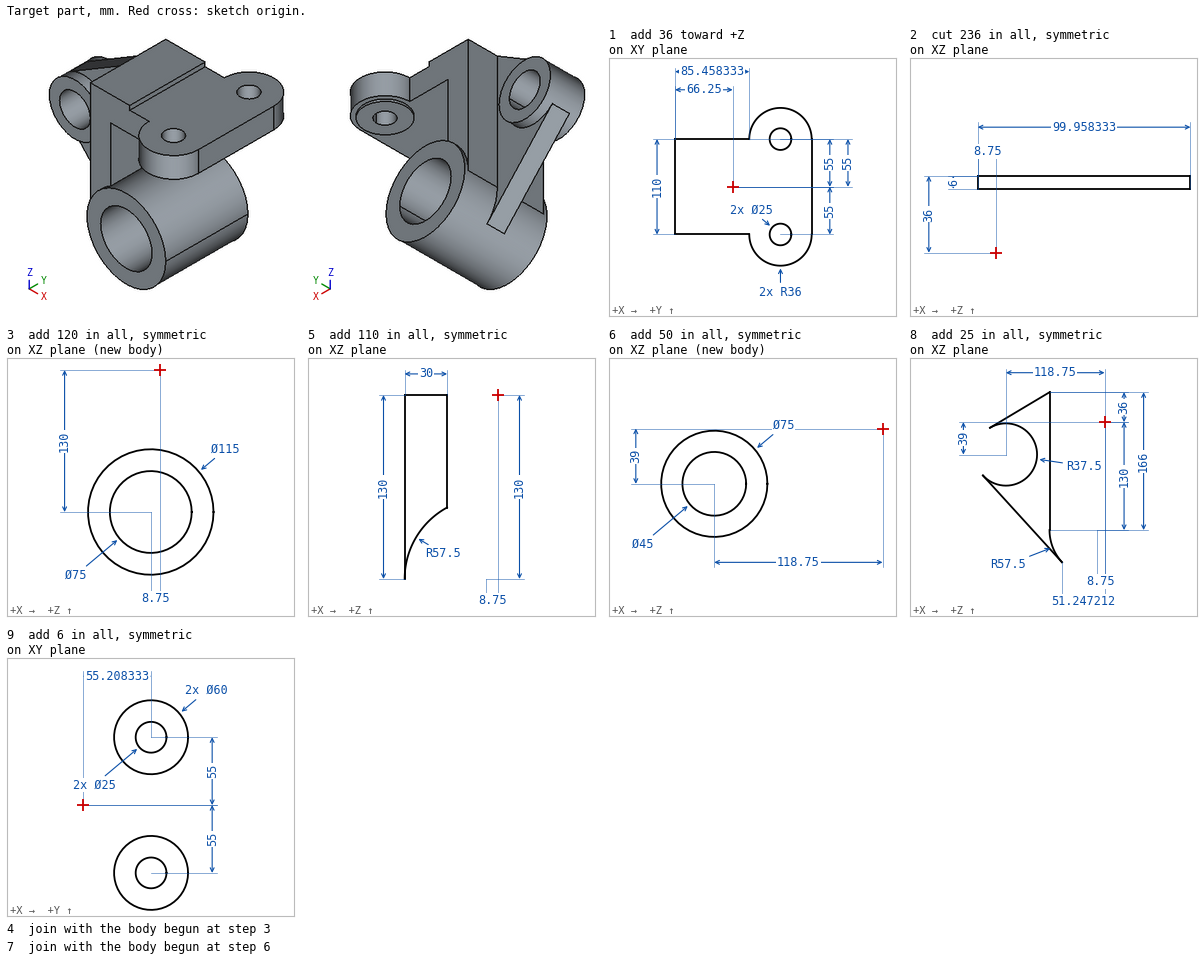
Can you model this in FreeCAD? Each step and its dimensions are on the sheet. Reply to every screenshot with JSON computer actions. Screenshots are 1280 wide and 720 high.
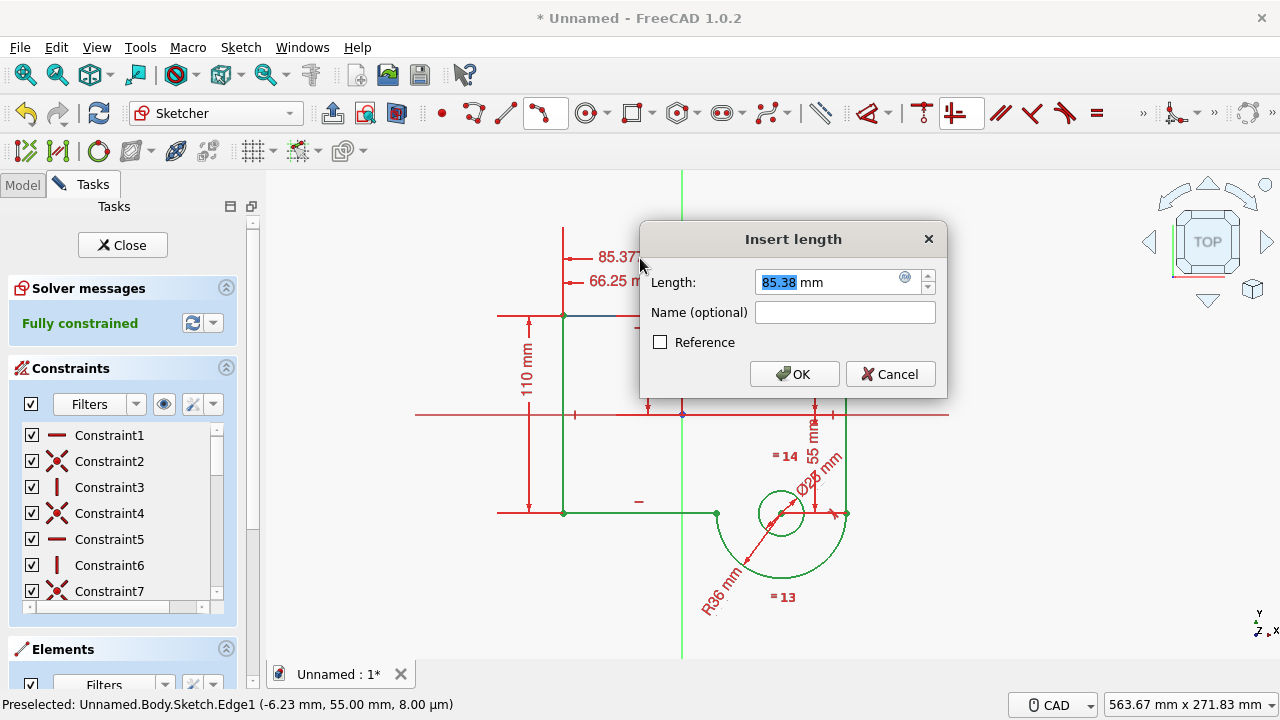
{"action": "type", "text": "85.458333"}
{"action": "key", "text": "Return"}
{"action": "key", "text": "Escape"}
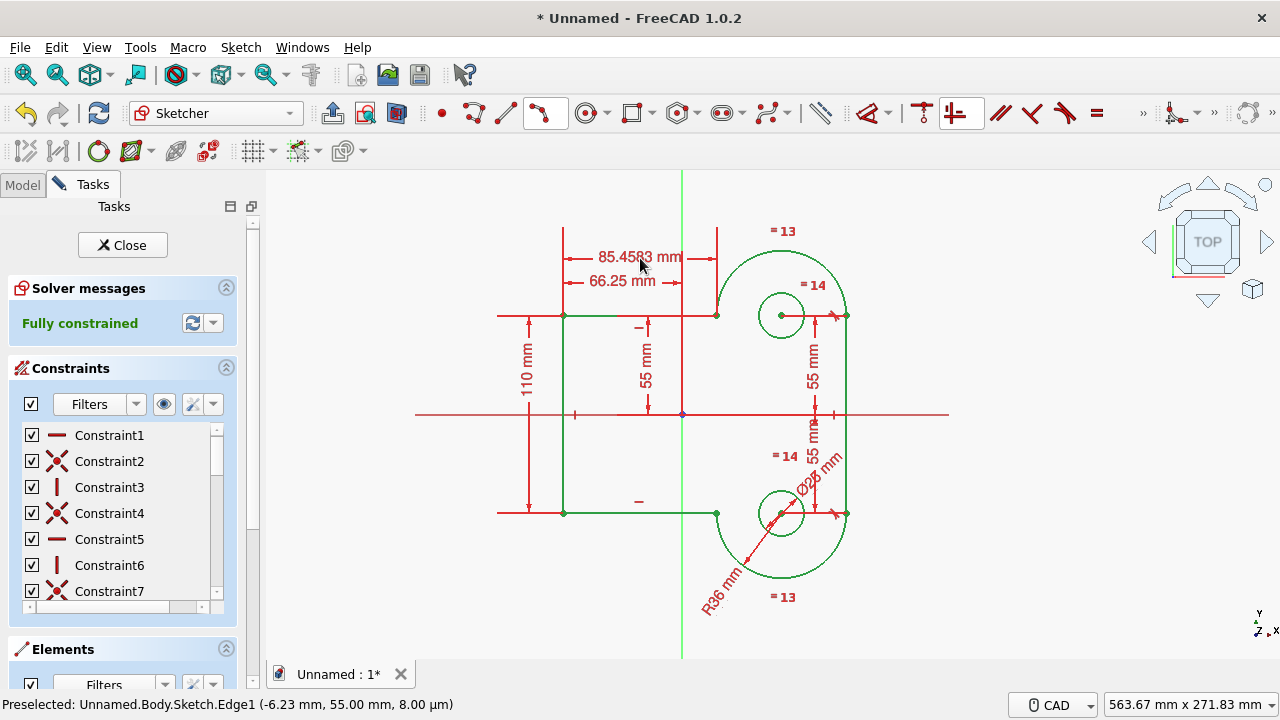
{"action": "left_click", "coordinate": [123, 245]}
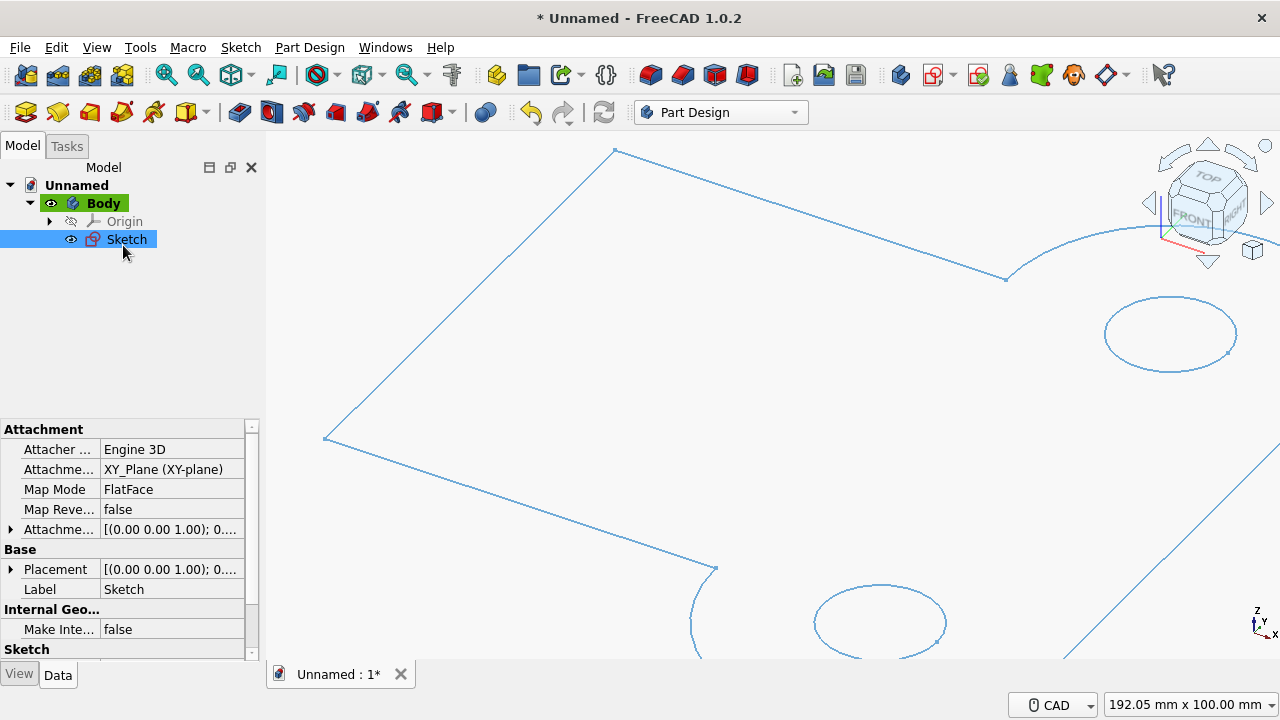
{"action": "left_click", "coordinate": [26, 112]}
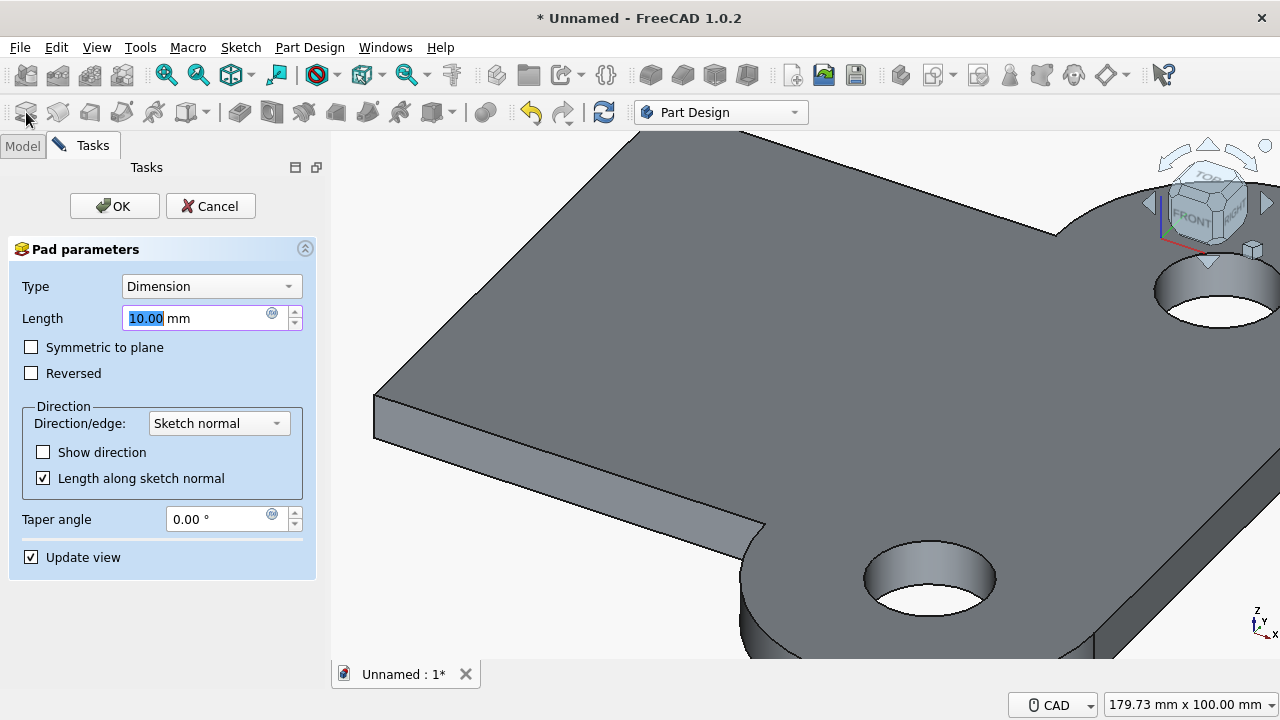
{"action": "type", "text": "36"}
{"action": "key", "text": "Tab"}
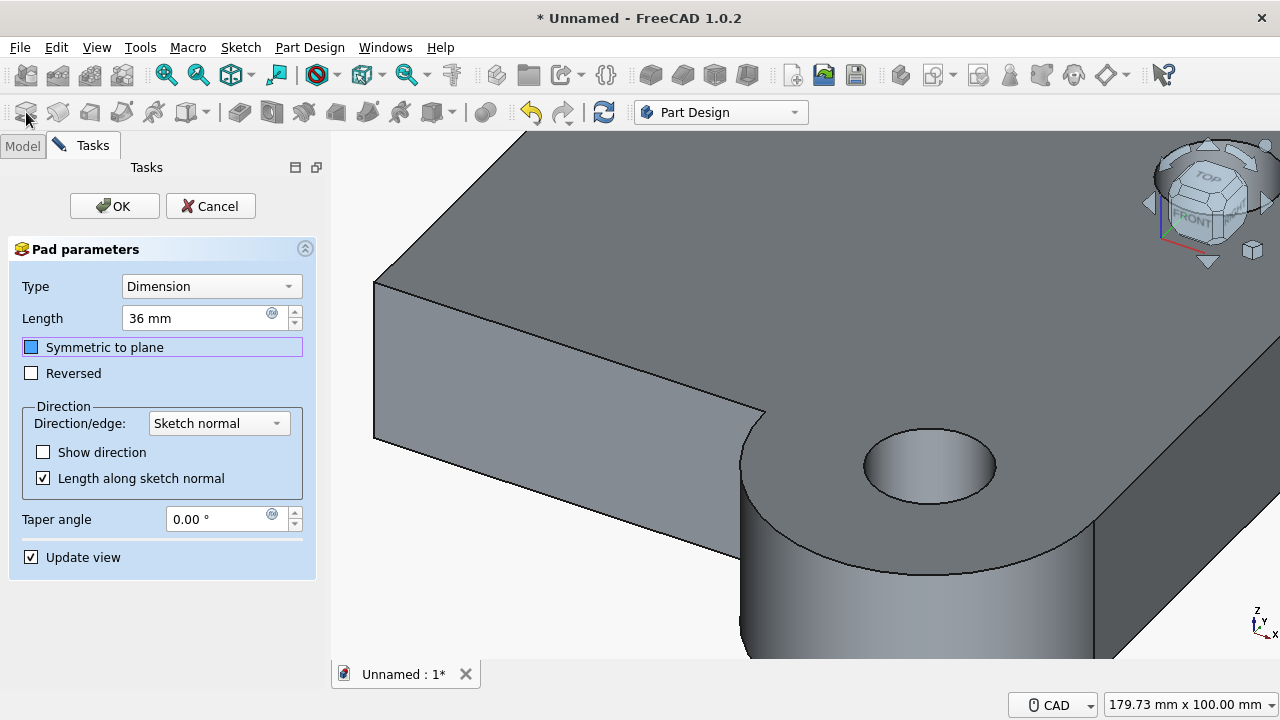
{"action": "left_click", "coordinate": [115, 206]}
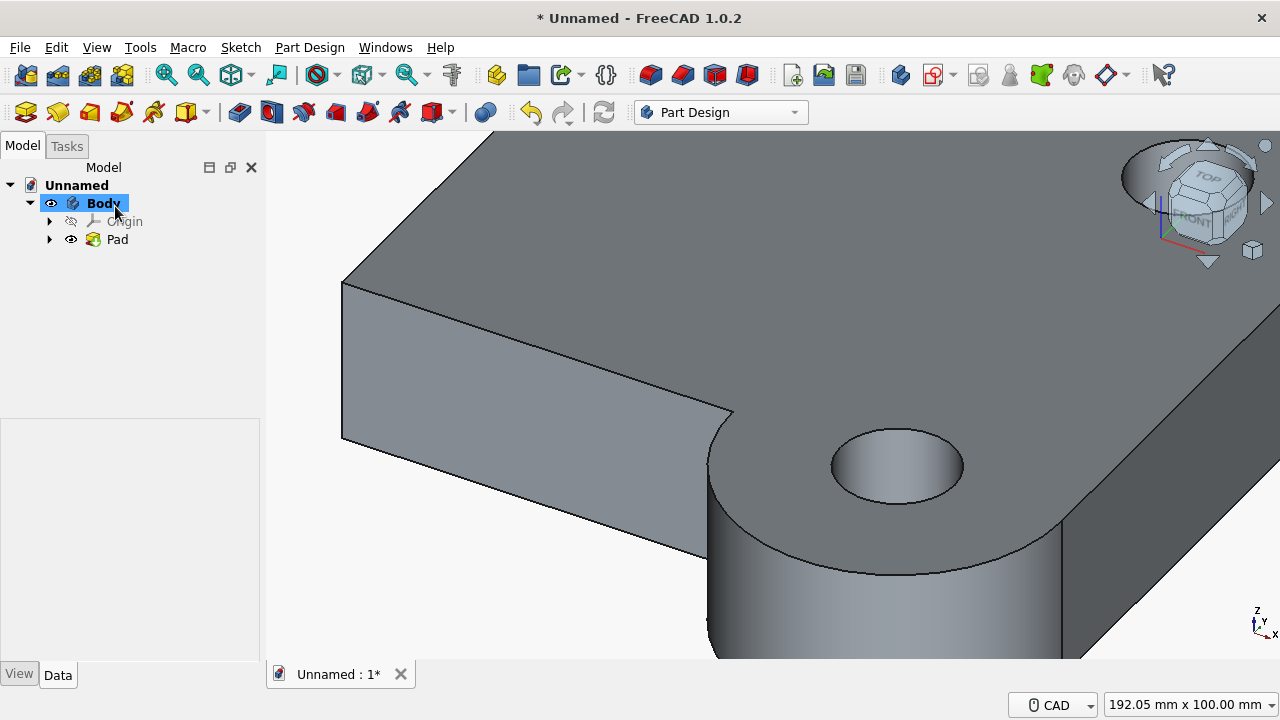
{"action": "left_click", "coordinate": [168, 76]}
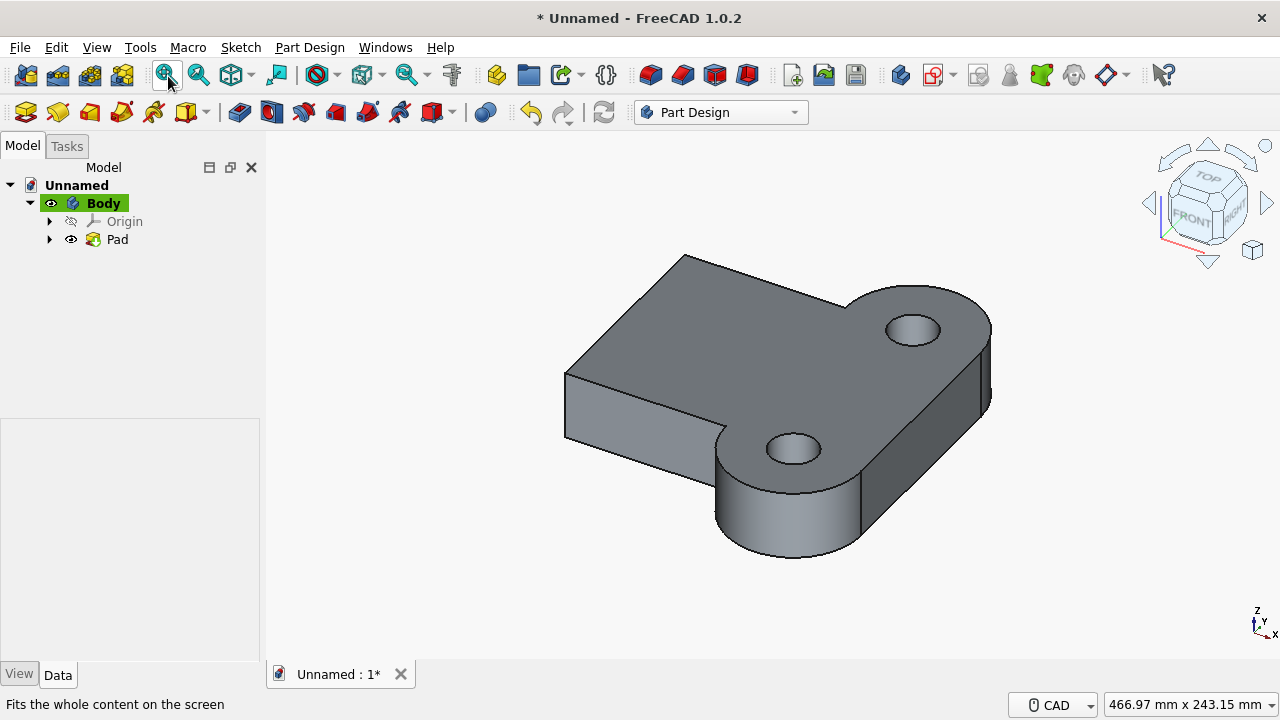
{"action": "left_click", "coordinate": [934, 76]}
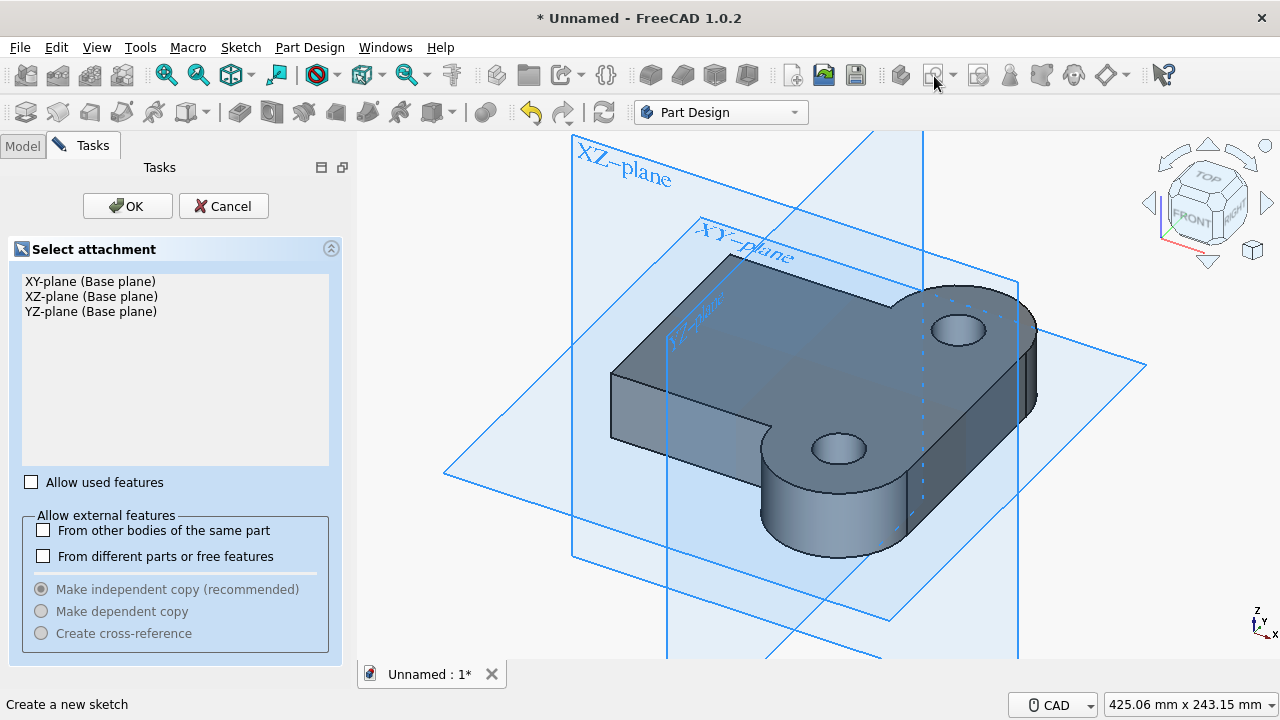
{"action": "left_click", "coordinate": [82, 296]}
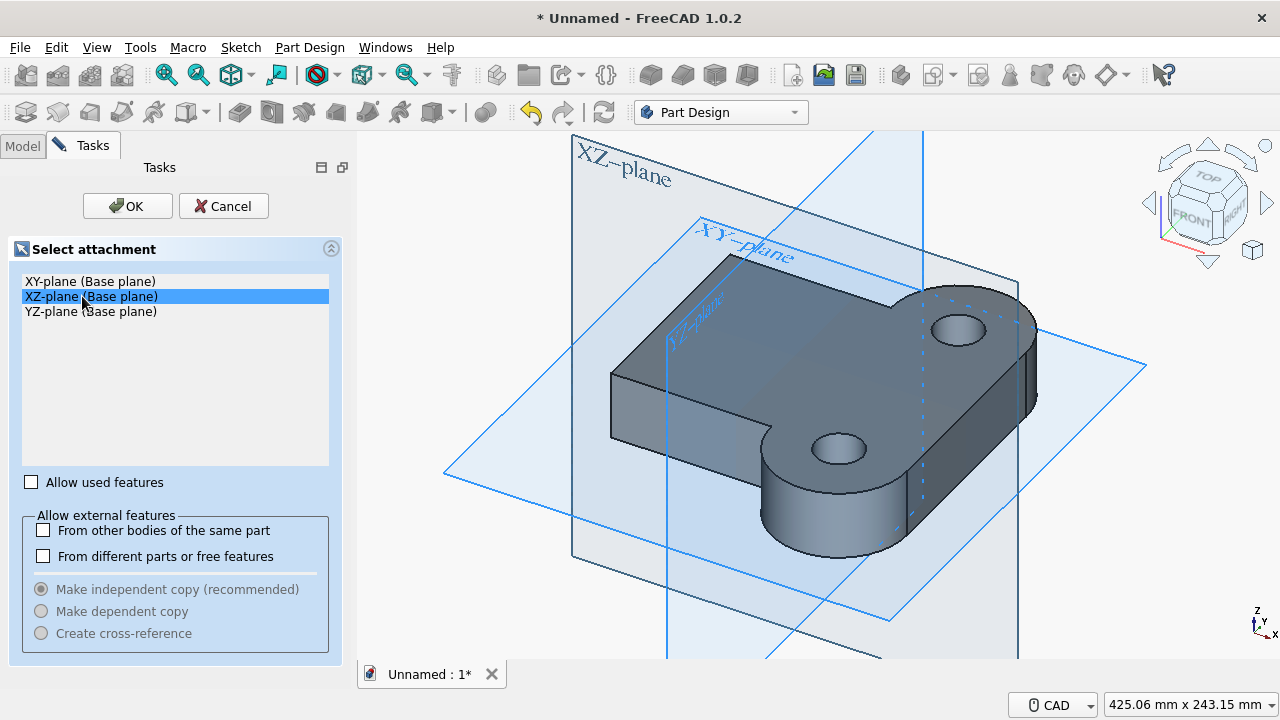
{"action": "left_click", "coordinate": [128, 206]}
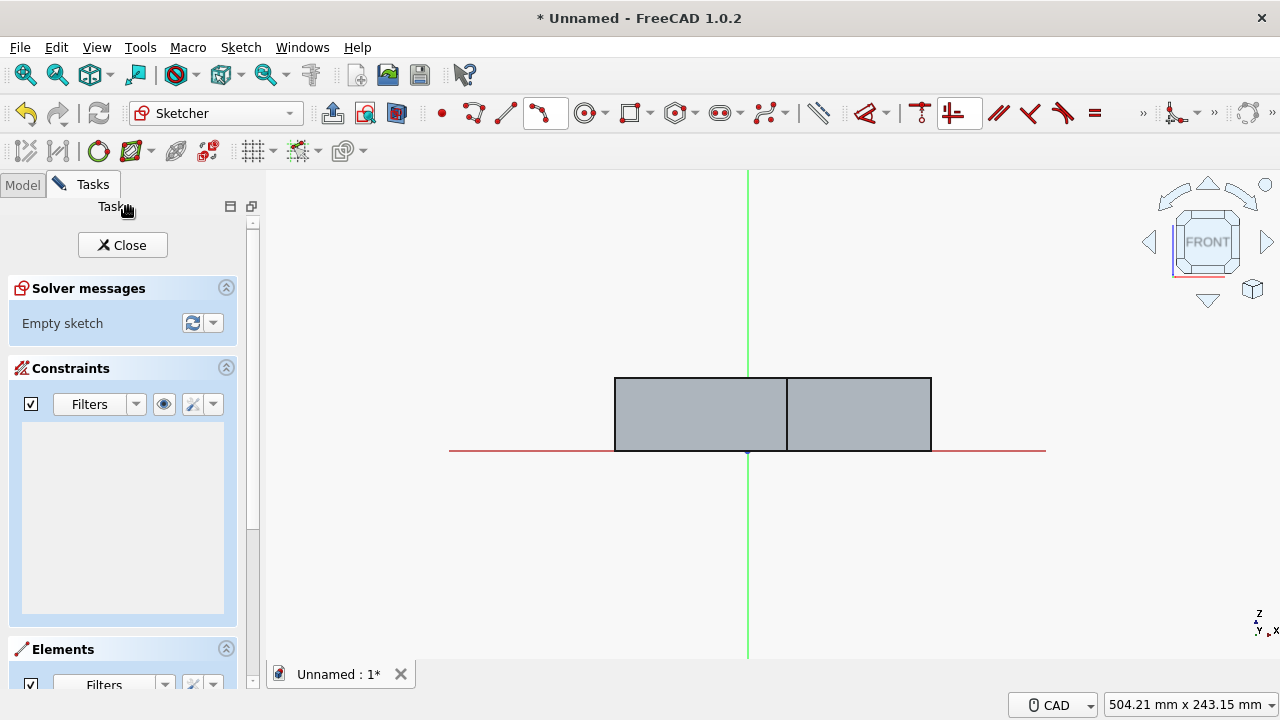
{"action": "left_click", "coordinate": [398, 114]}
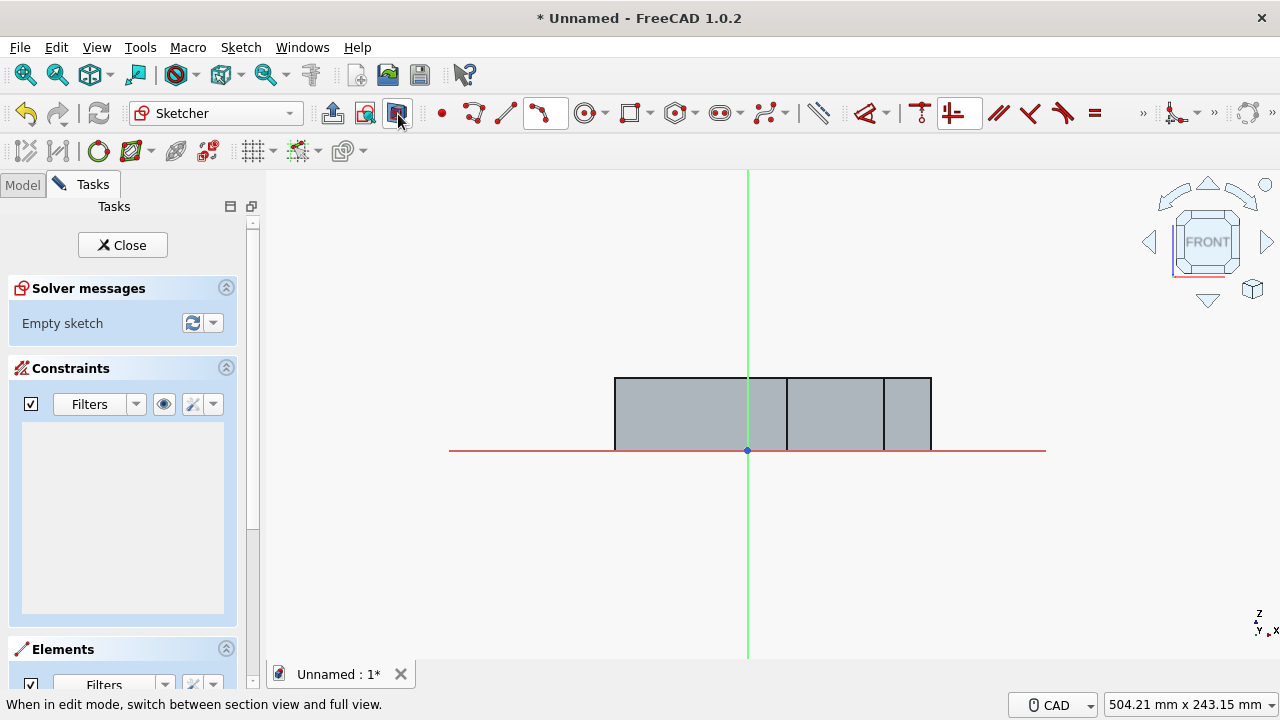
{"action": "scroll", "coordinate": [904, 415], "scroll_direction": "up", "scroll_amount": 5}